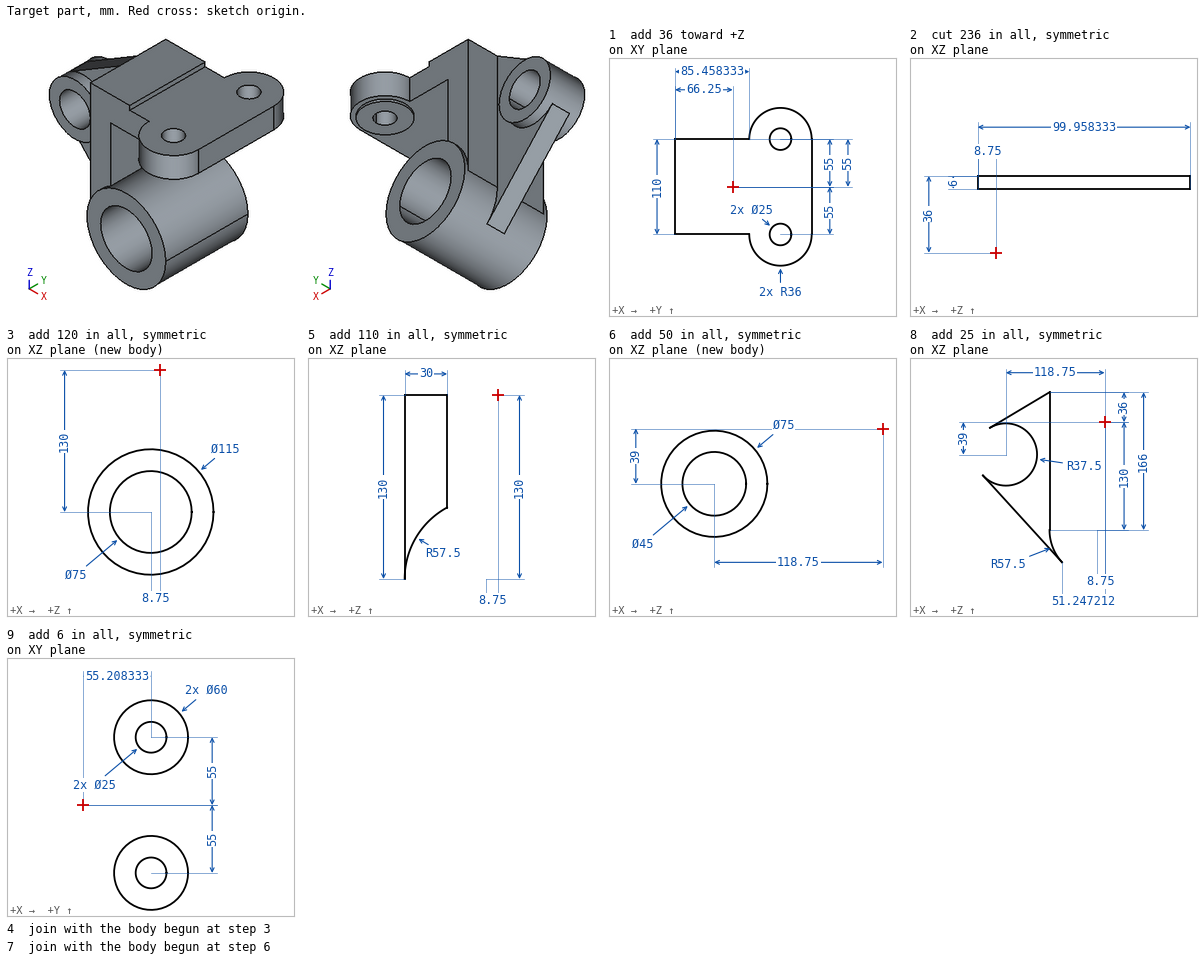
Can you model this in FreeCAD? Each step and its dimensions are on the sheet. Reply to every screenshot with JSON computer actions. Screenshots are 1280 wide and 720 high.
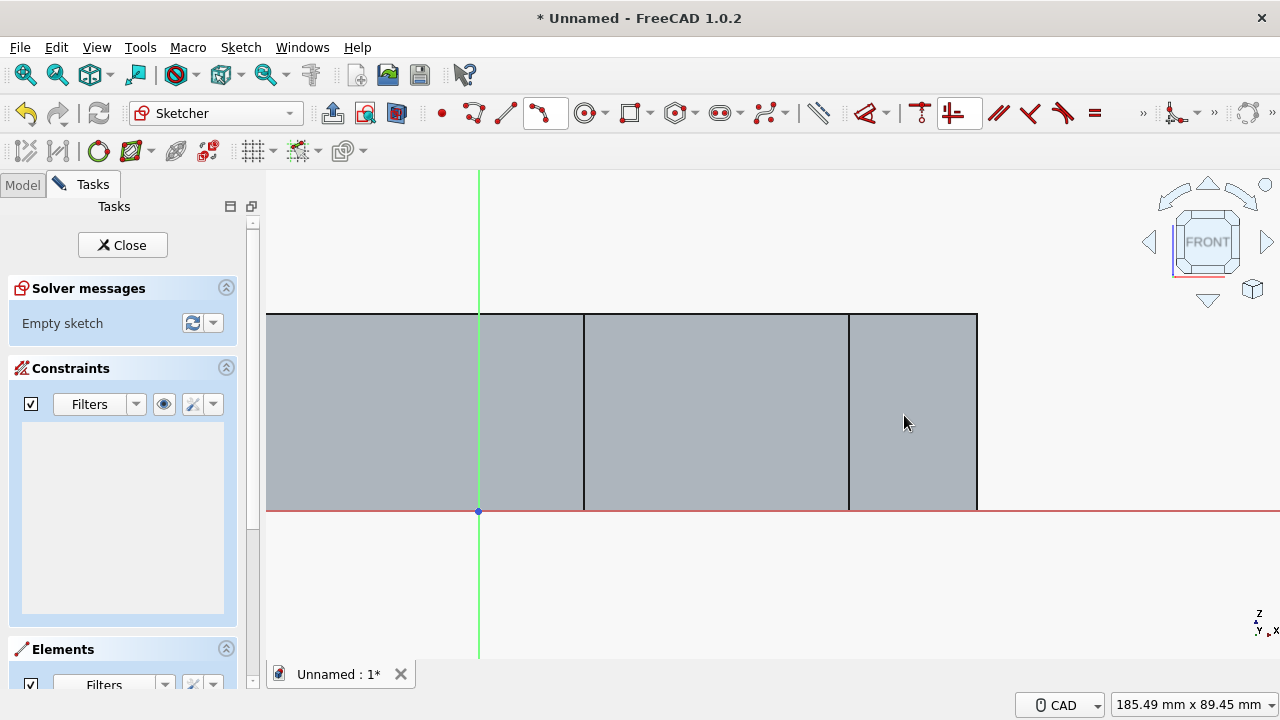
{"action": "left_click", "coordinate": [630, 114]}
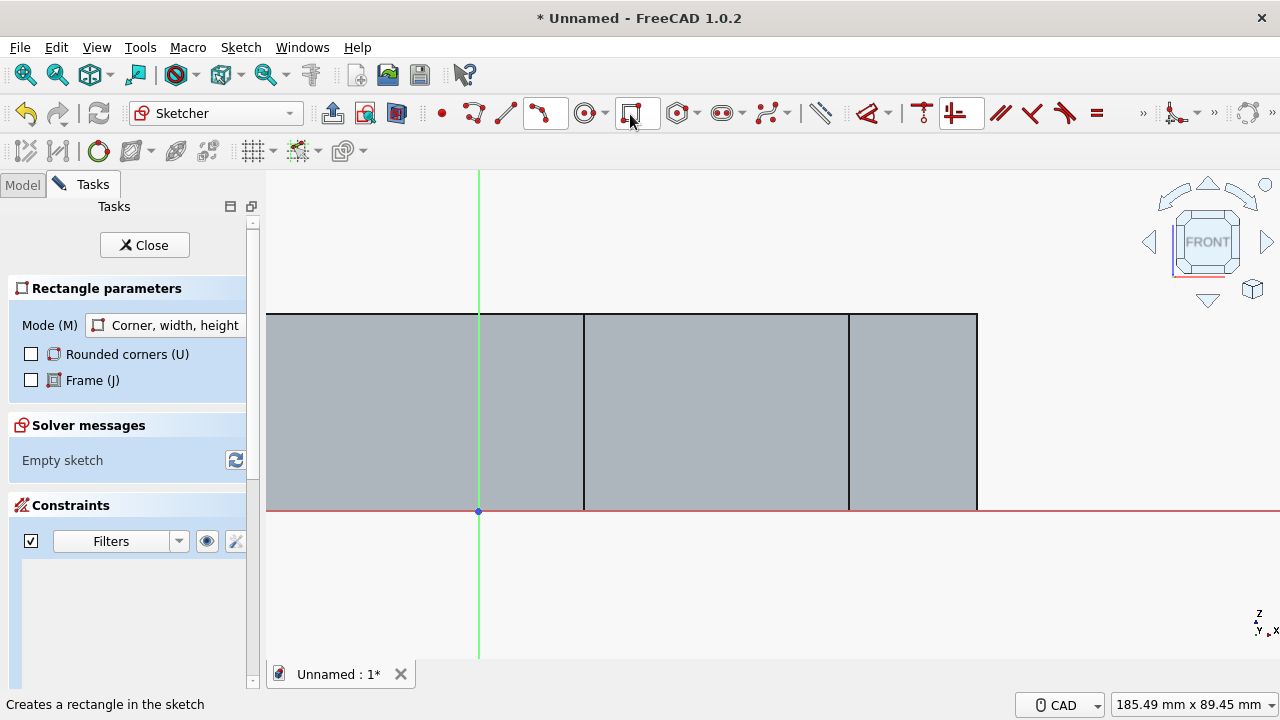
{"action": "left_click", "coordinate": [431, 314]}
{"action": "left_click", "coordinate": [977, 347]}
{"action": "key", "text": "Escape"}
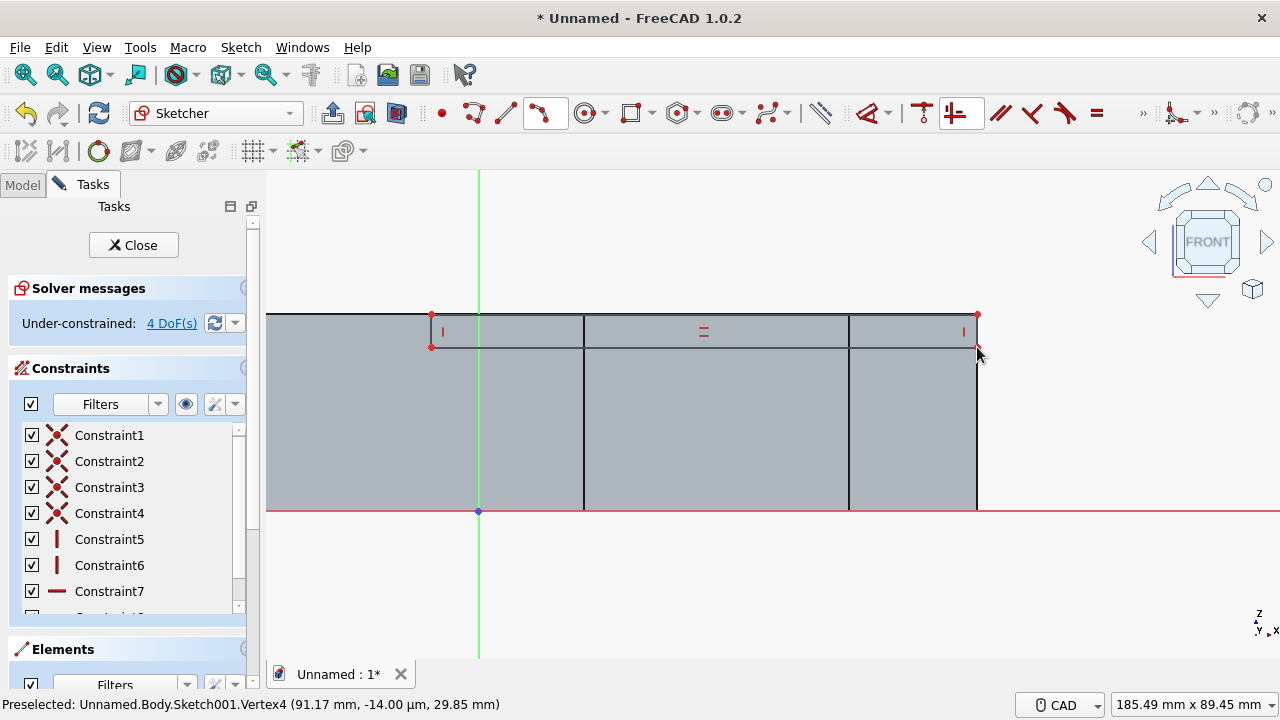
{"action": "left_click", "coordinate": [868, 114]}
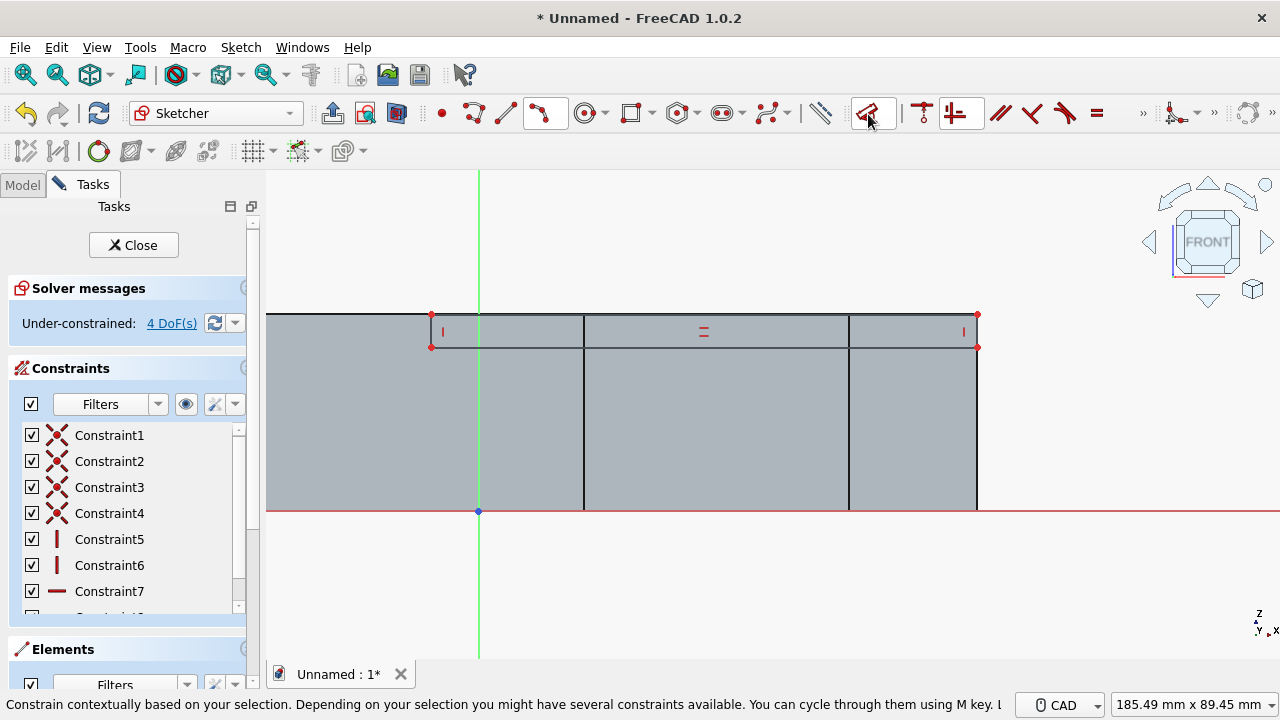
{"action": "scroll", "coordinate": [431, 325], "scroll_direction": "up", "scroll_amount": 2}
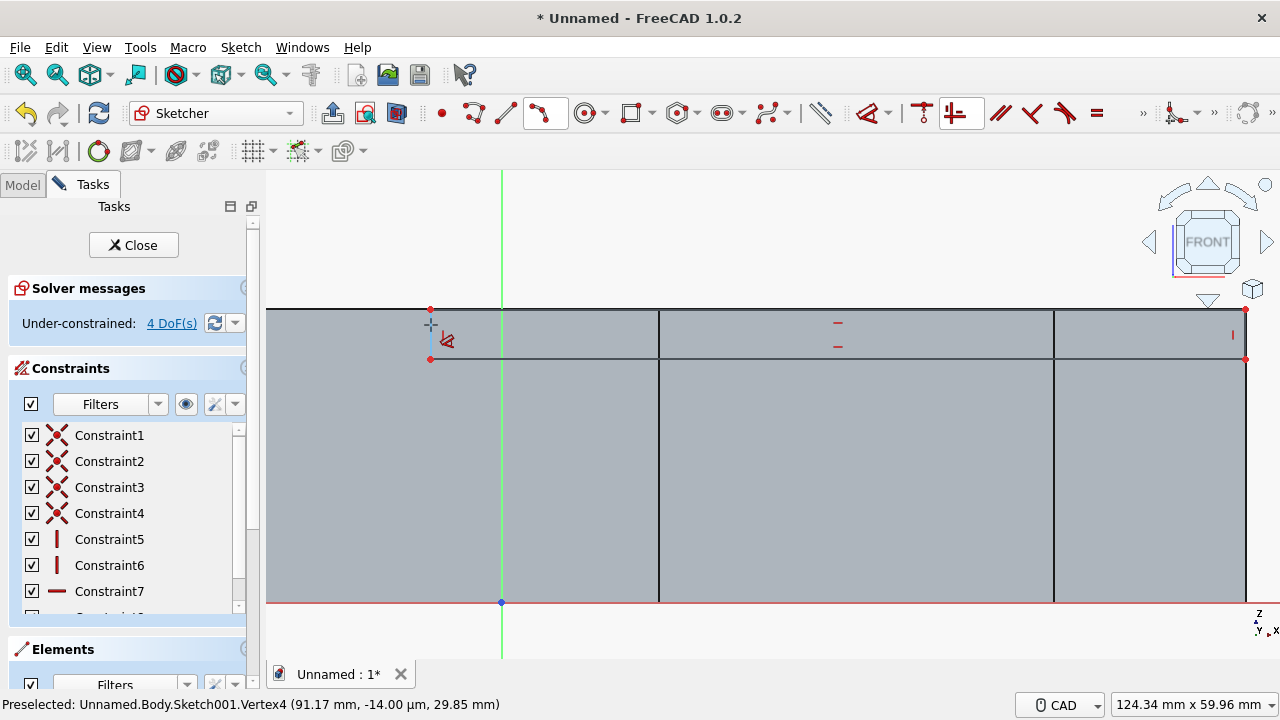
{"action": "left_click", "coordinate": [431, 325]}
{"action": "left_click", "coordinate": [397, 335]}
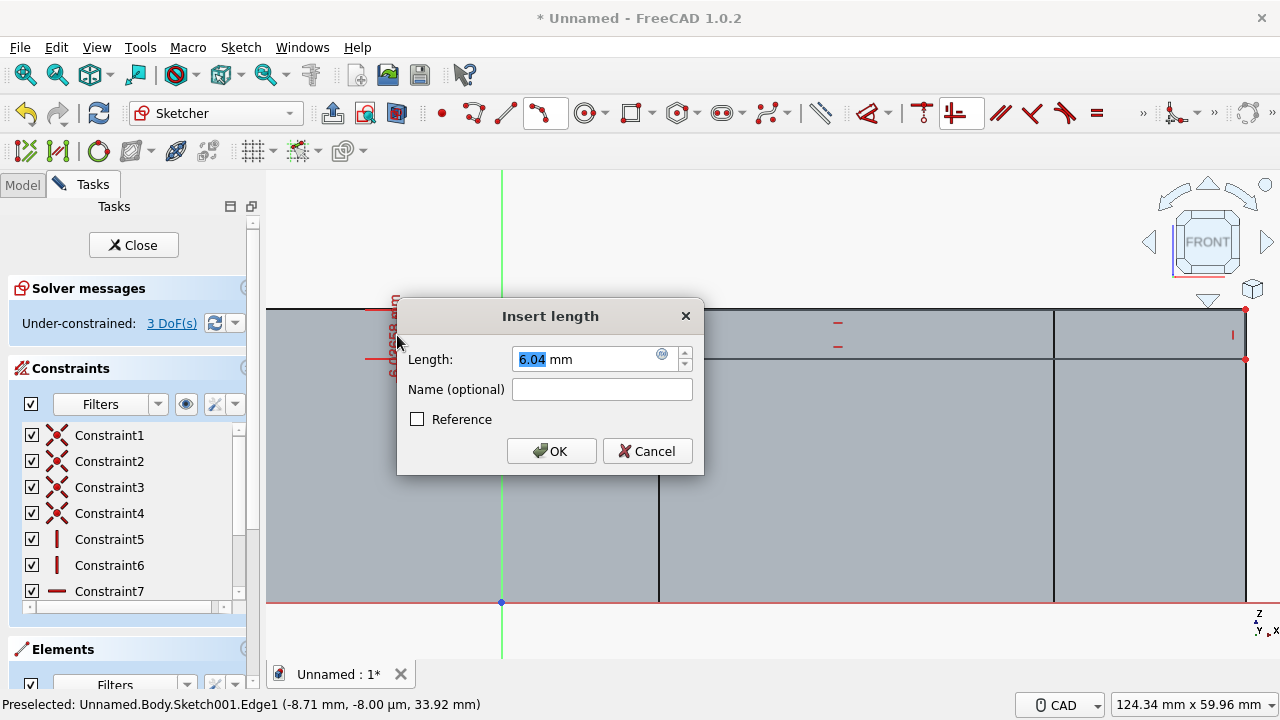
{"action": "type", "text": "6"}
{"action": "key", "text": "Return"}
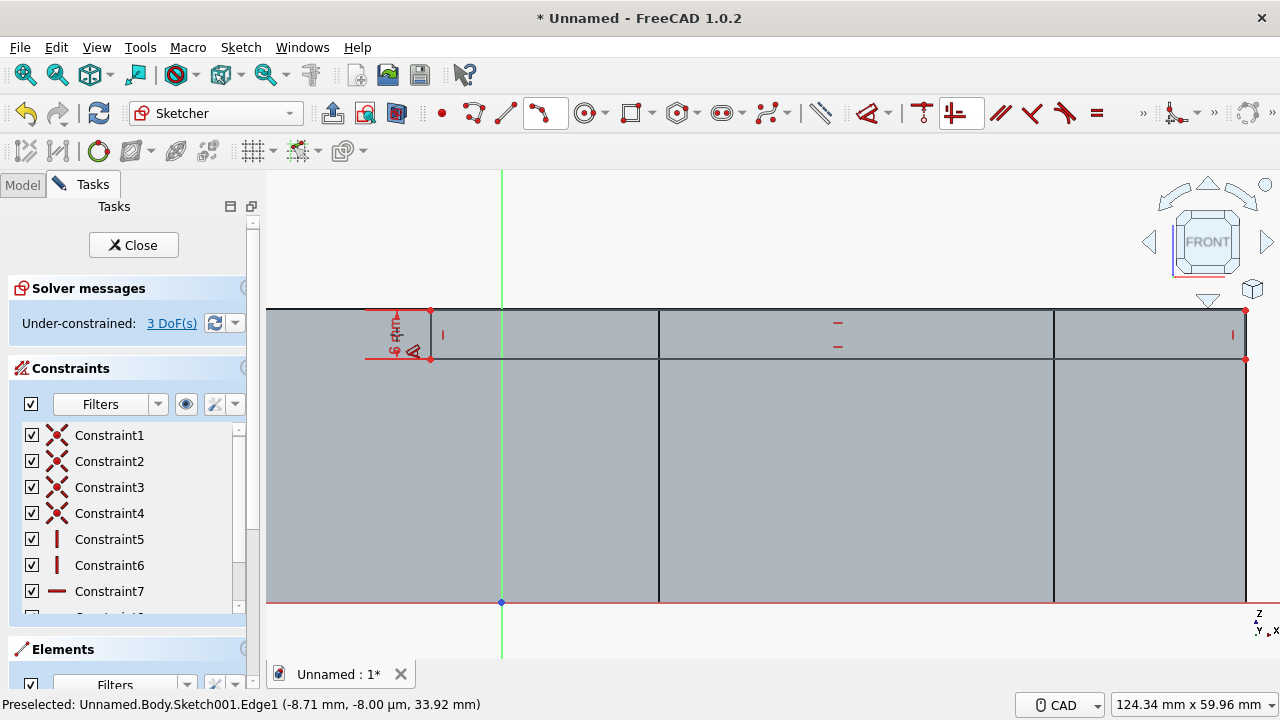
{"action": "left_click", "coordinate": [431, 310]}
{"action": "left_click", "coordinate": [397, 456]}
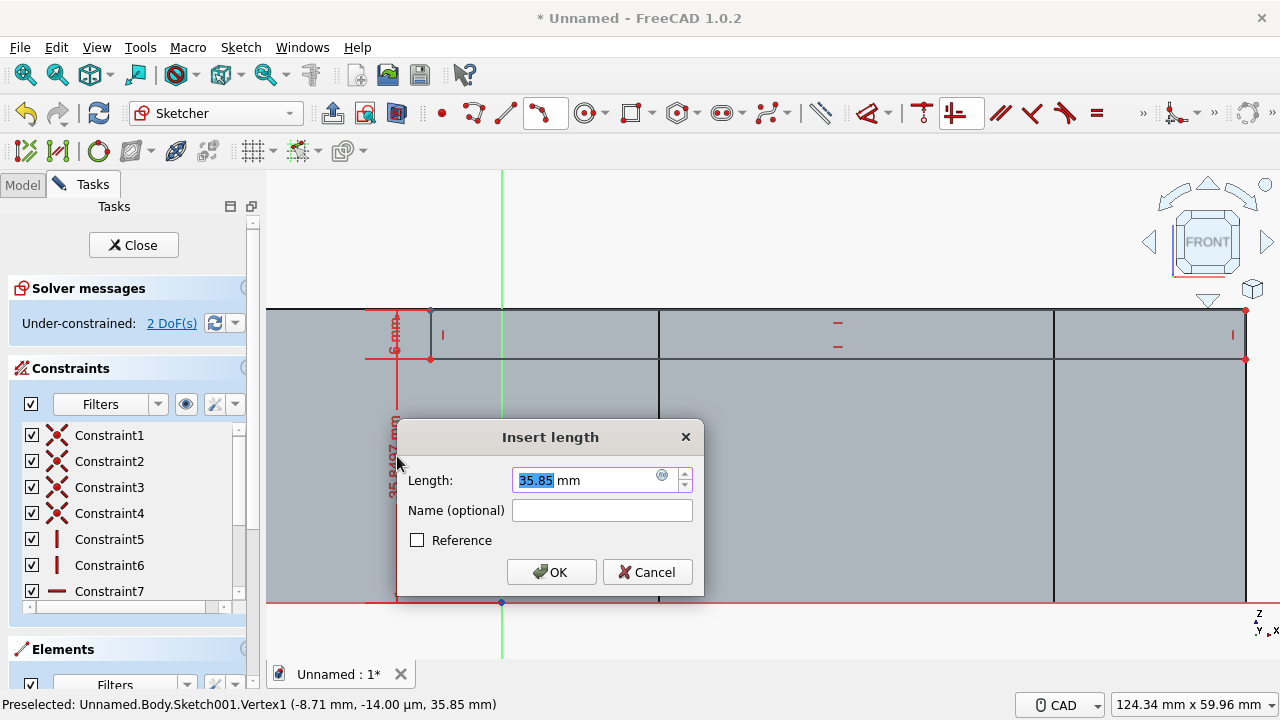
{"action": "type", "text": "36"}
{"action": "key", "text": "Return"}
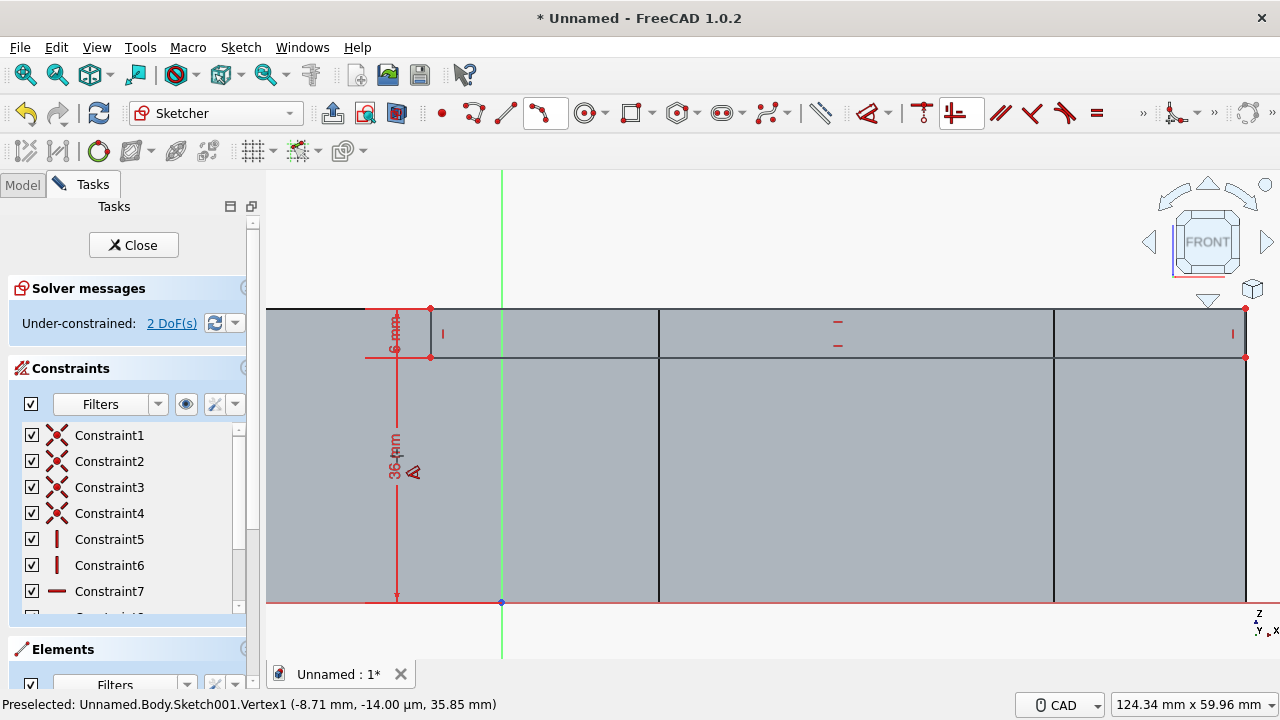
{"action": "left_click", "coordinate": [431, 309]}
{"action": "left_click", "coordinate": [466, 275]}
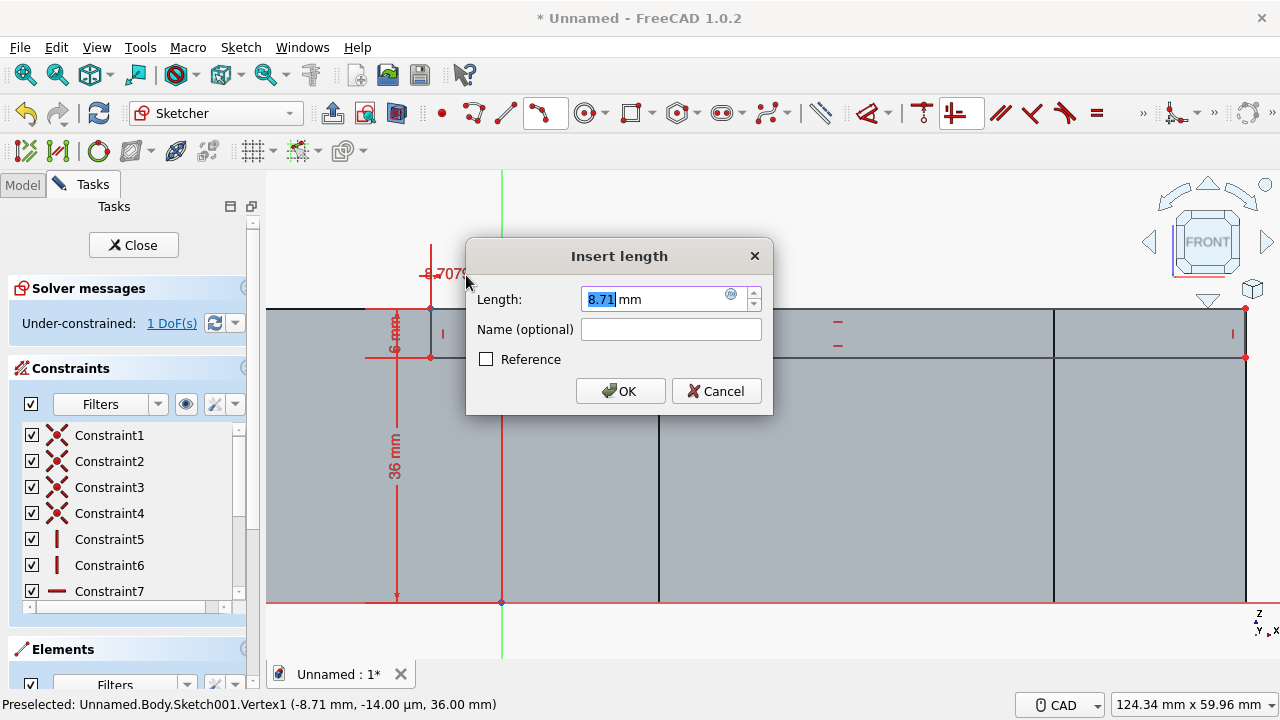
{"action": "type", "text": "8.75"}
{"action": "key", "text": "Return"}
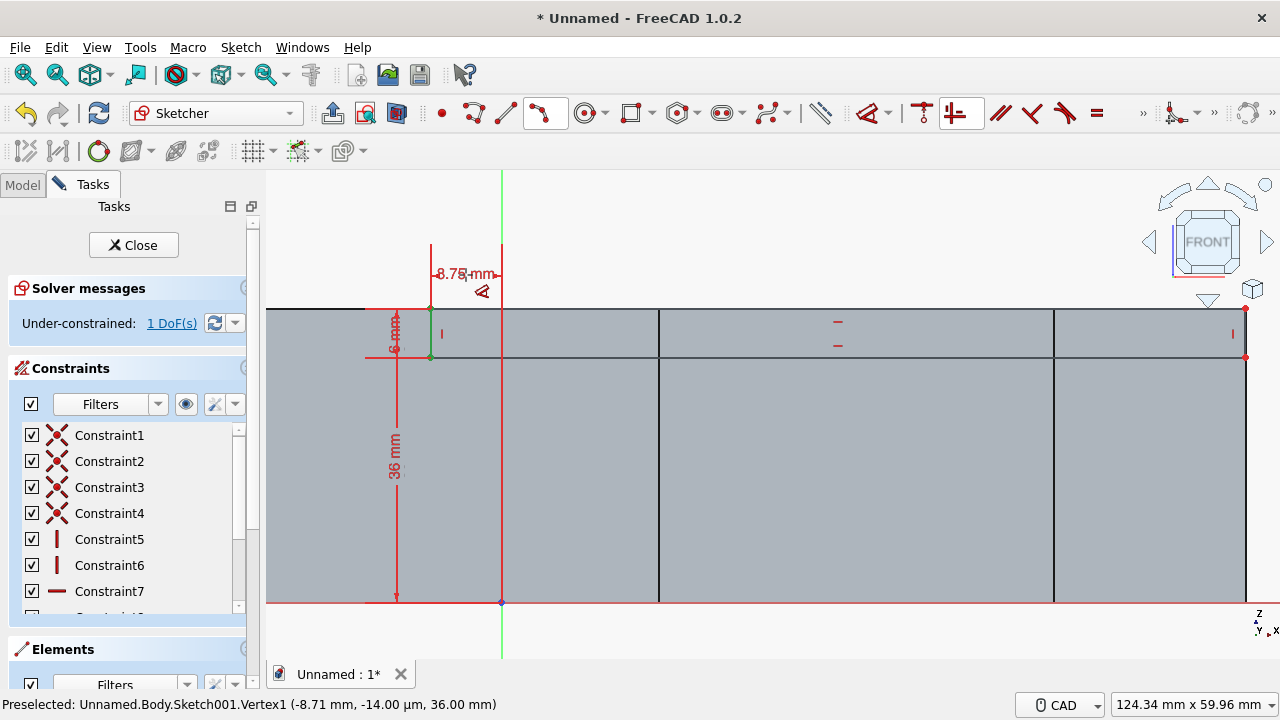
{"action": "left_click", "coordinate": [675, 358]}
{"action": "left_click", "coordinate": [773, 324]}